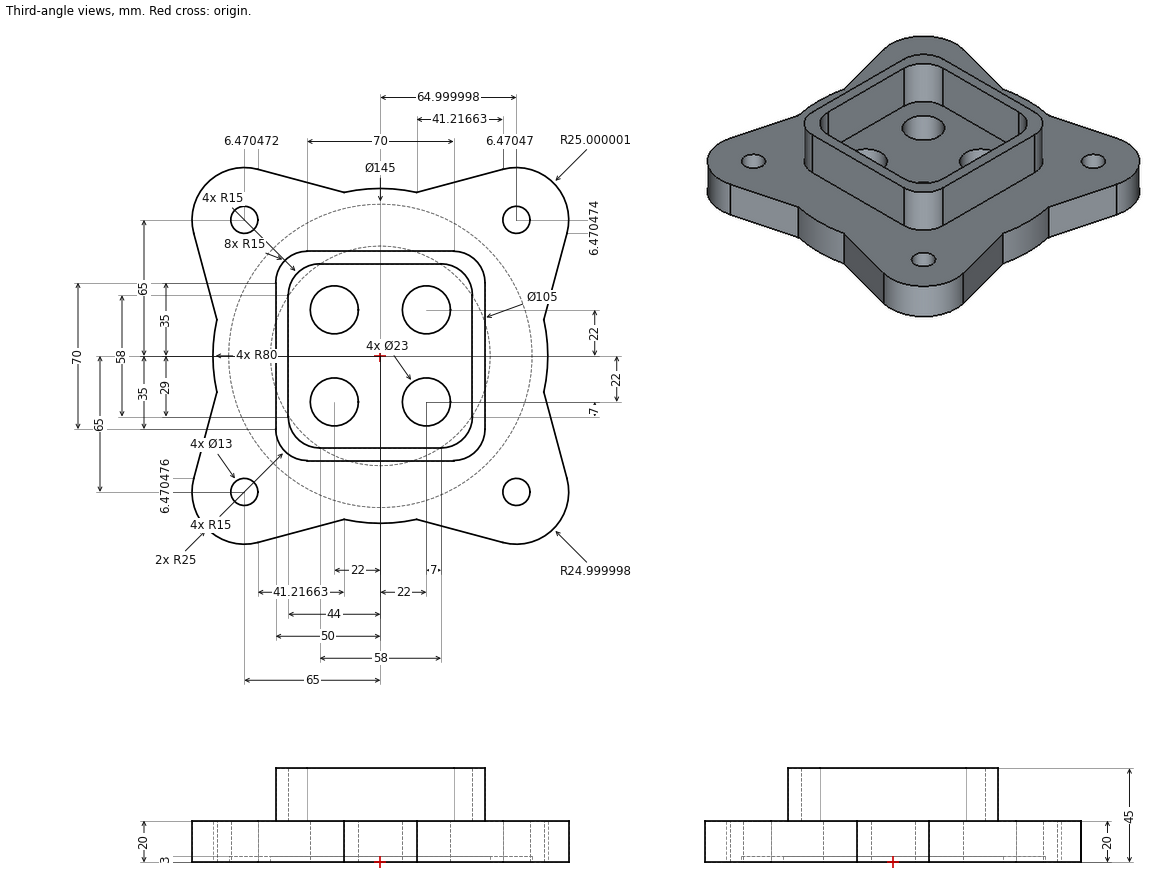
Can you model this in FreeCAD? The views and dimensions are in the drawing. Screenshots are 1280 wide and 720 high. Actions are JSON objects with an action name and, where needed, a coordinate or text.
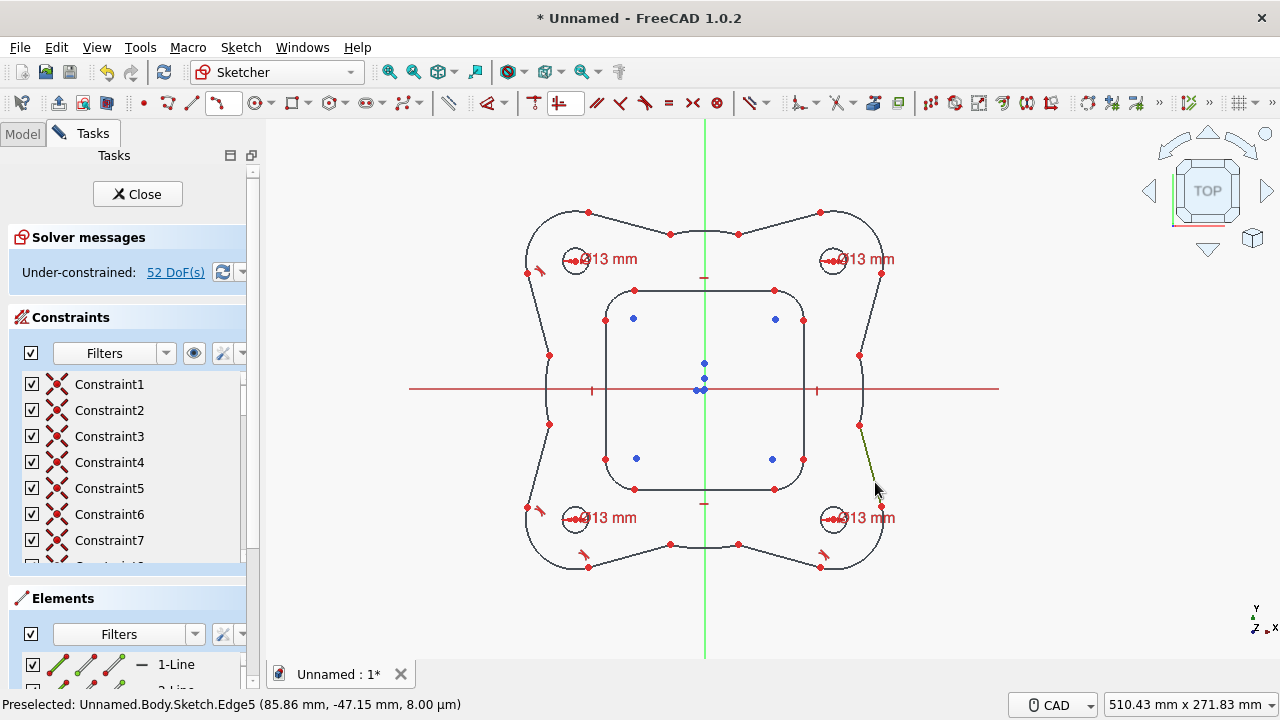
{"action": "left_click", "coordinate": [851, 566]}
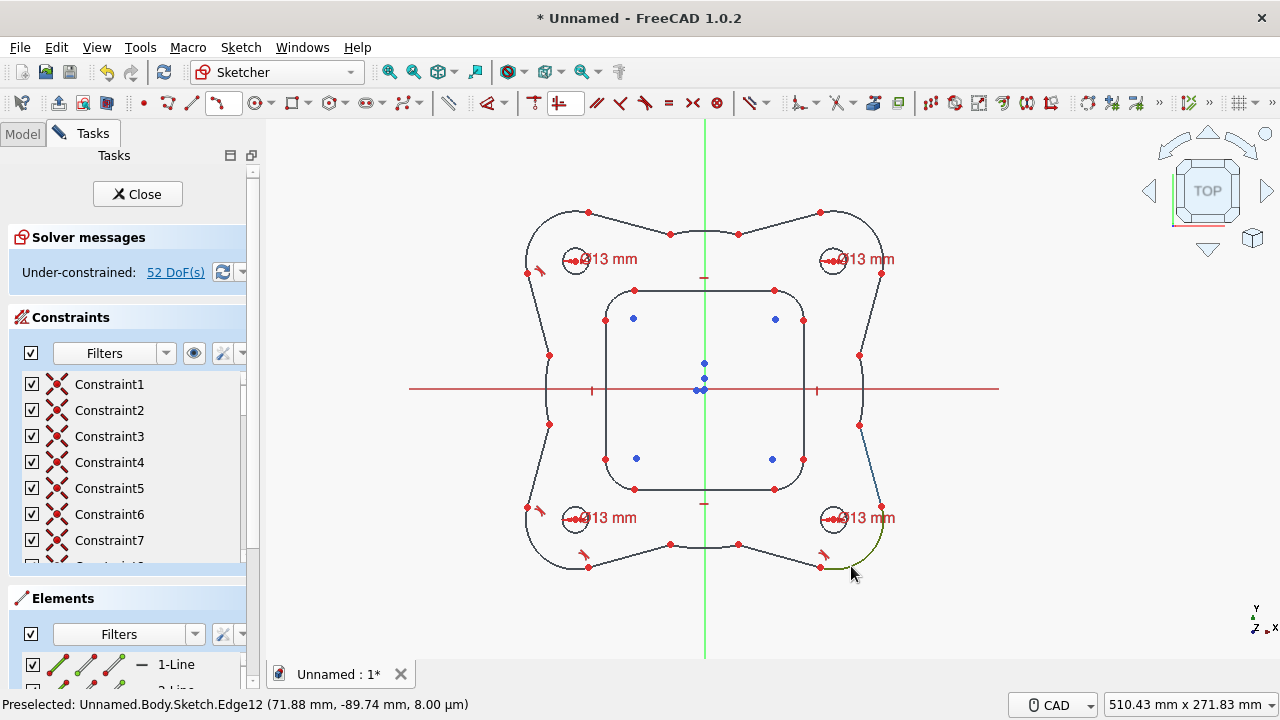
{"action": "left_click", "coordinate": [646, 104]}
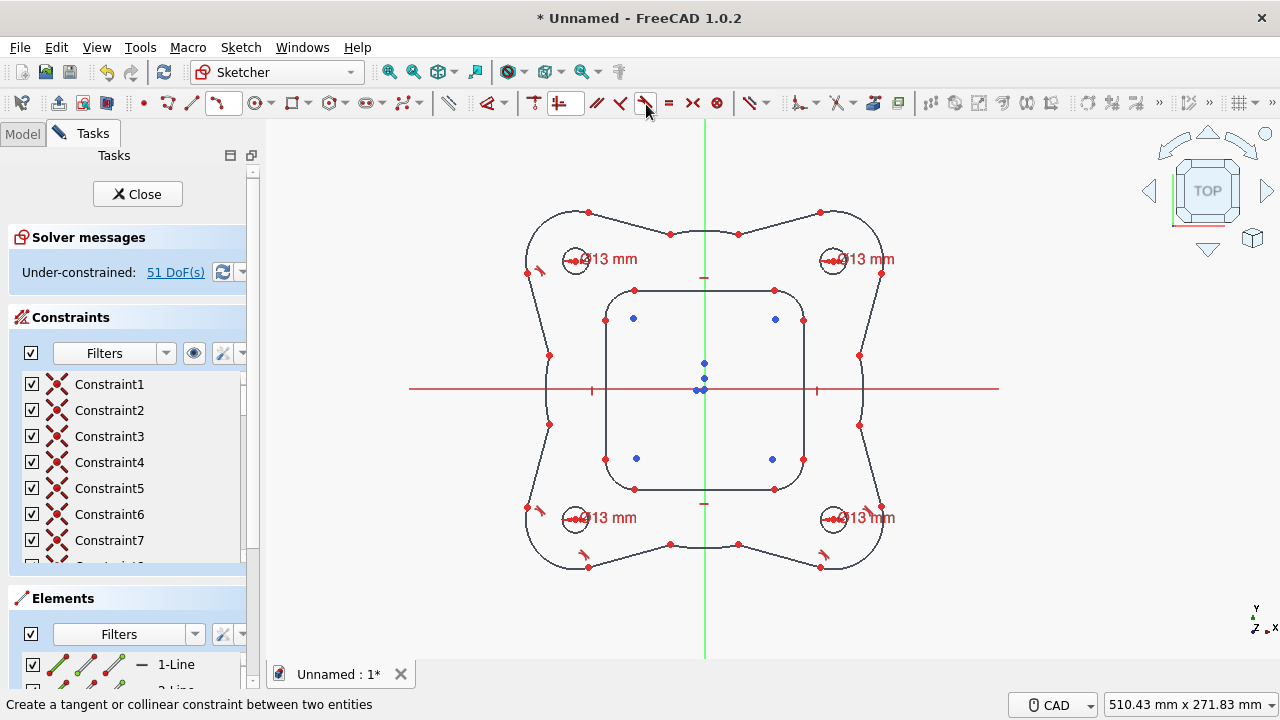
{"action": "left_click", "coordinate": [866, 331]}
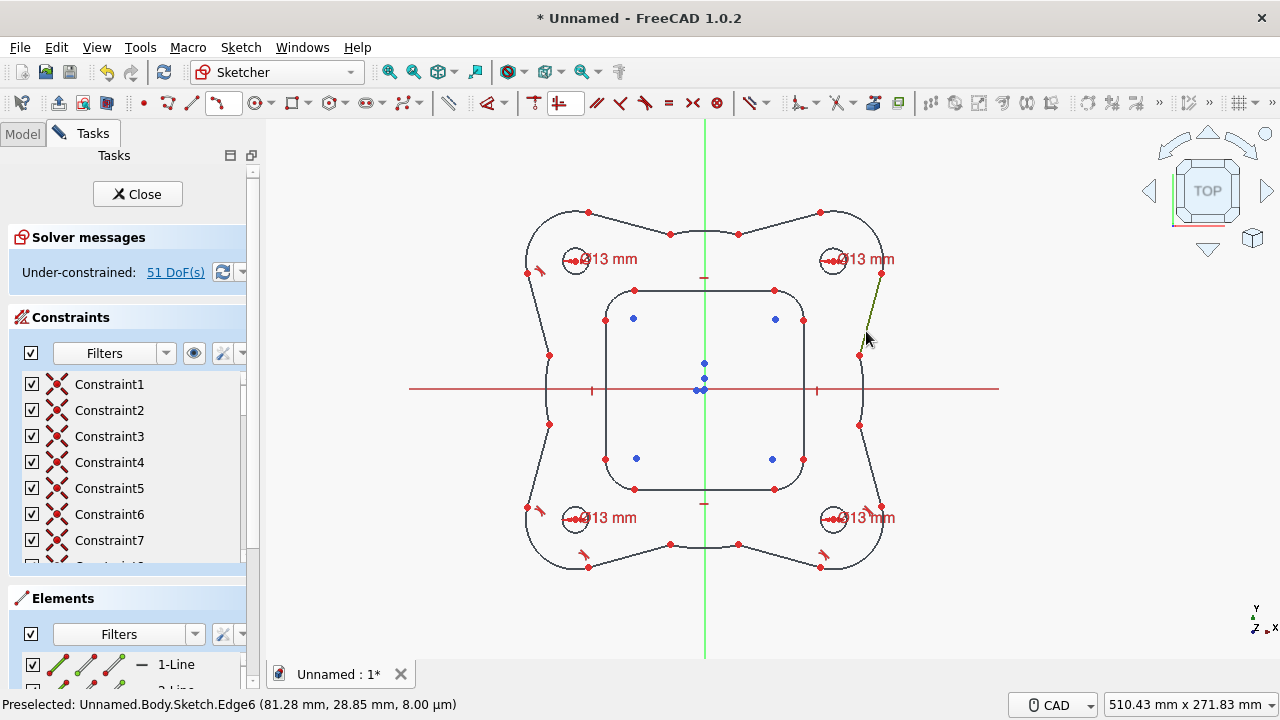
{"action": "left_click", "coordinate": [880, 243]}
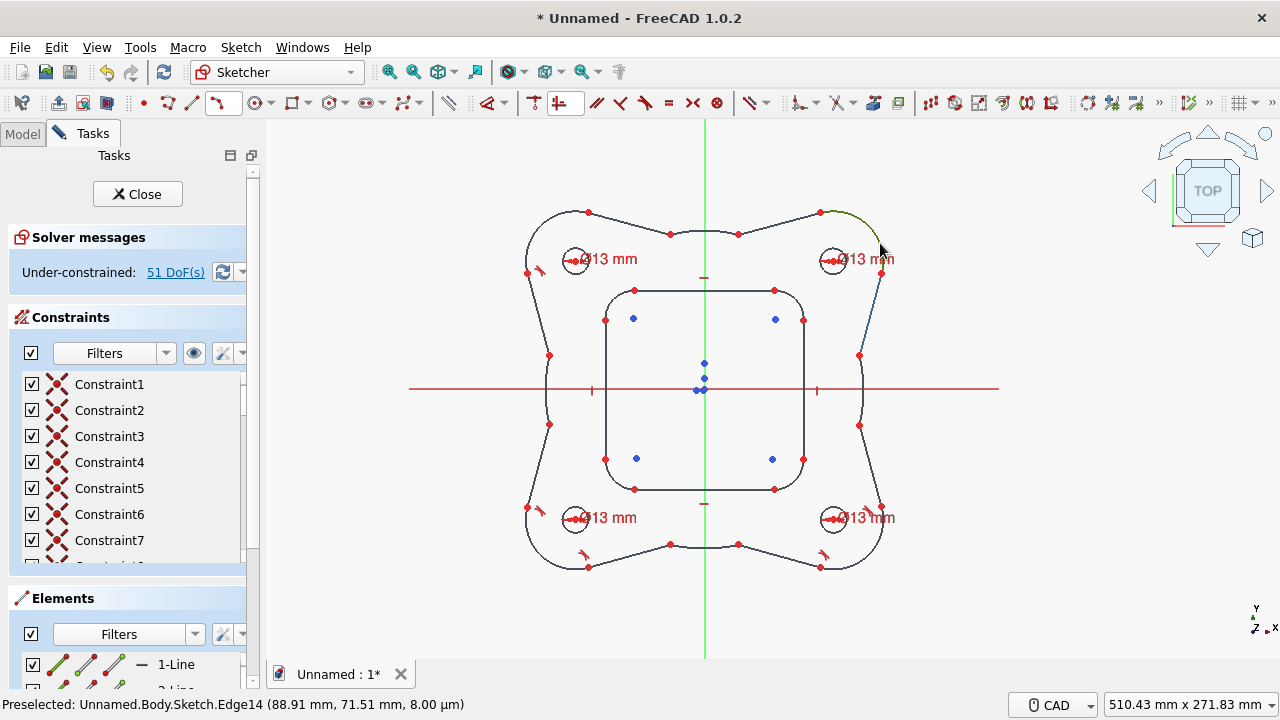
{"action": "left_click", "coordinate": [646, 104]}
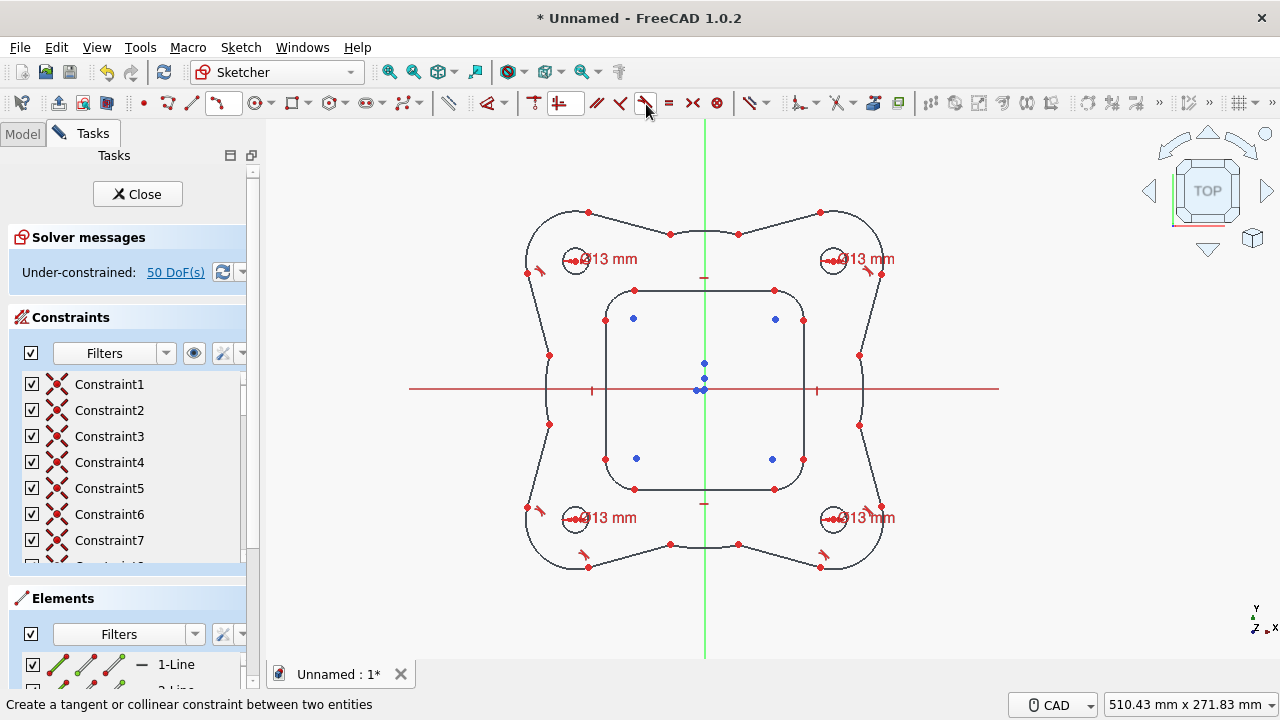
{"action": "left_click", "coordinate": [796, 220]}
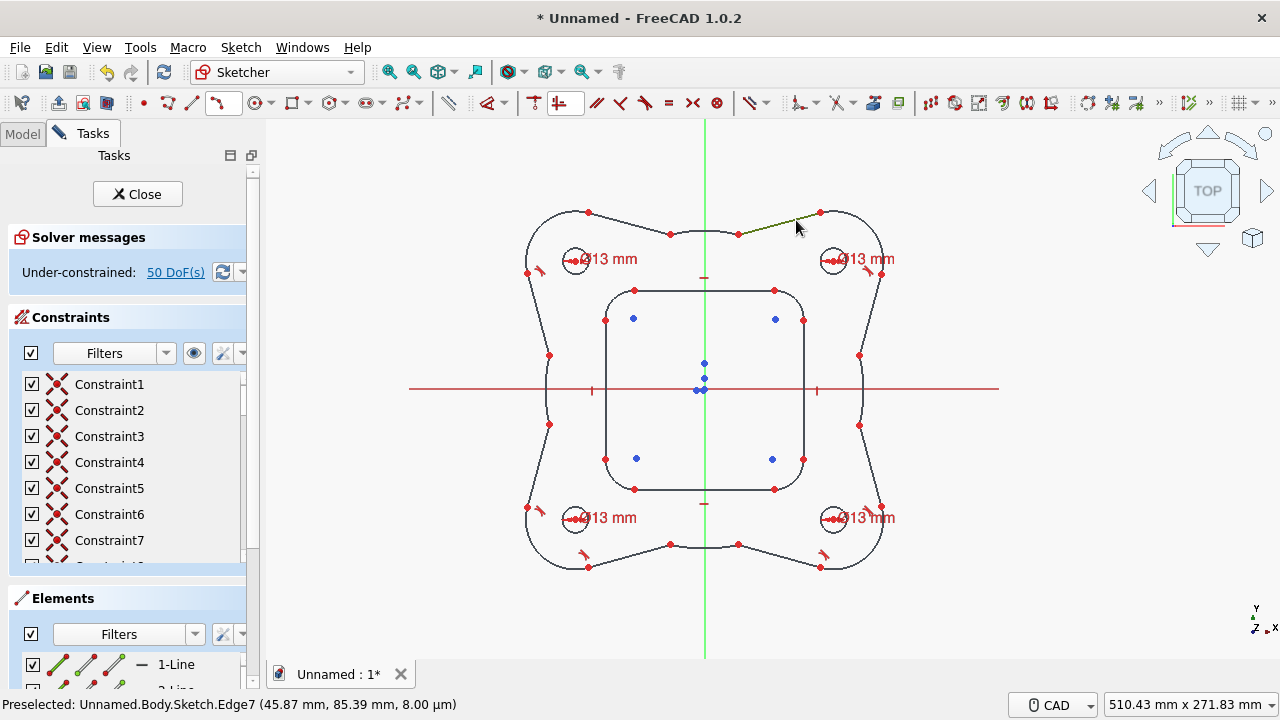
{"action": "left_click", "coordinate": [880, 243]}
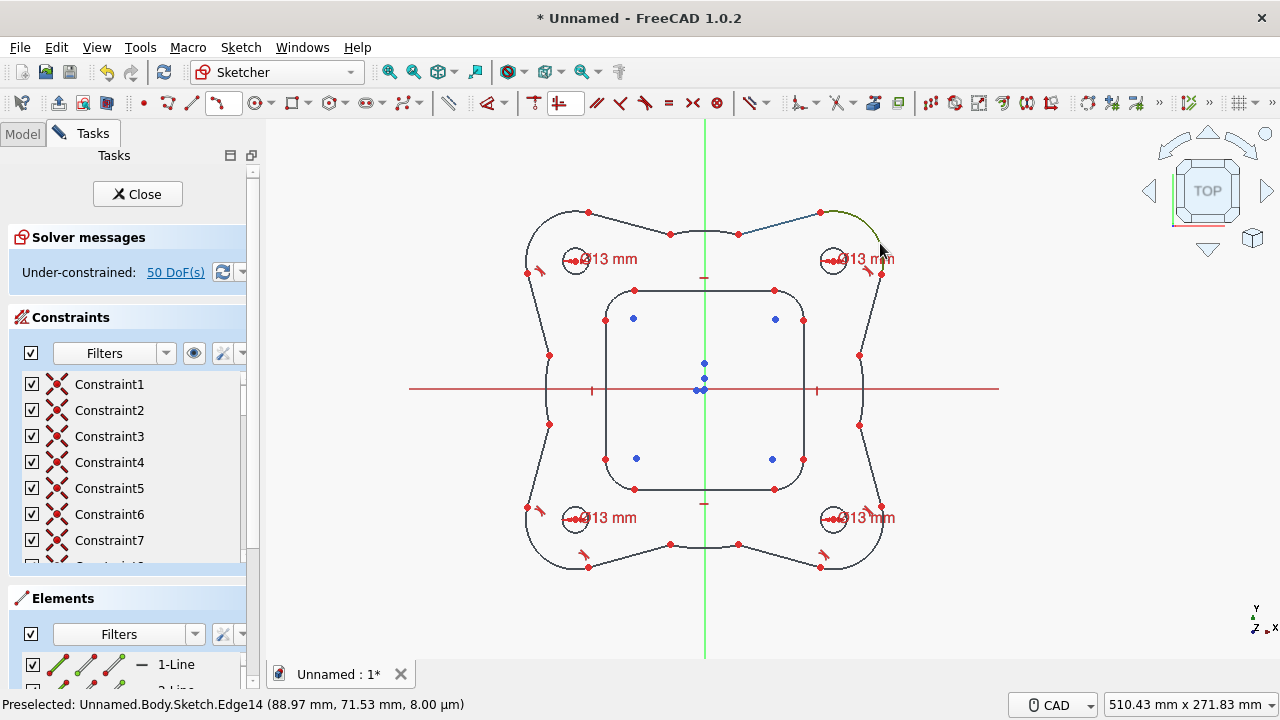
{"action": "left_click", "coordinate": [646, 104]}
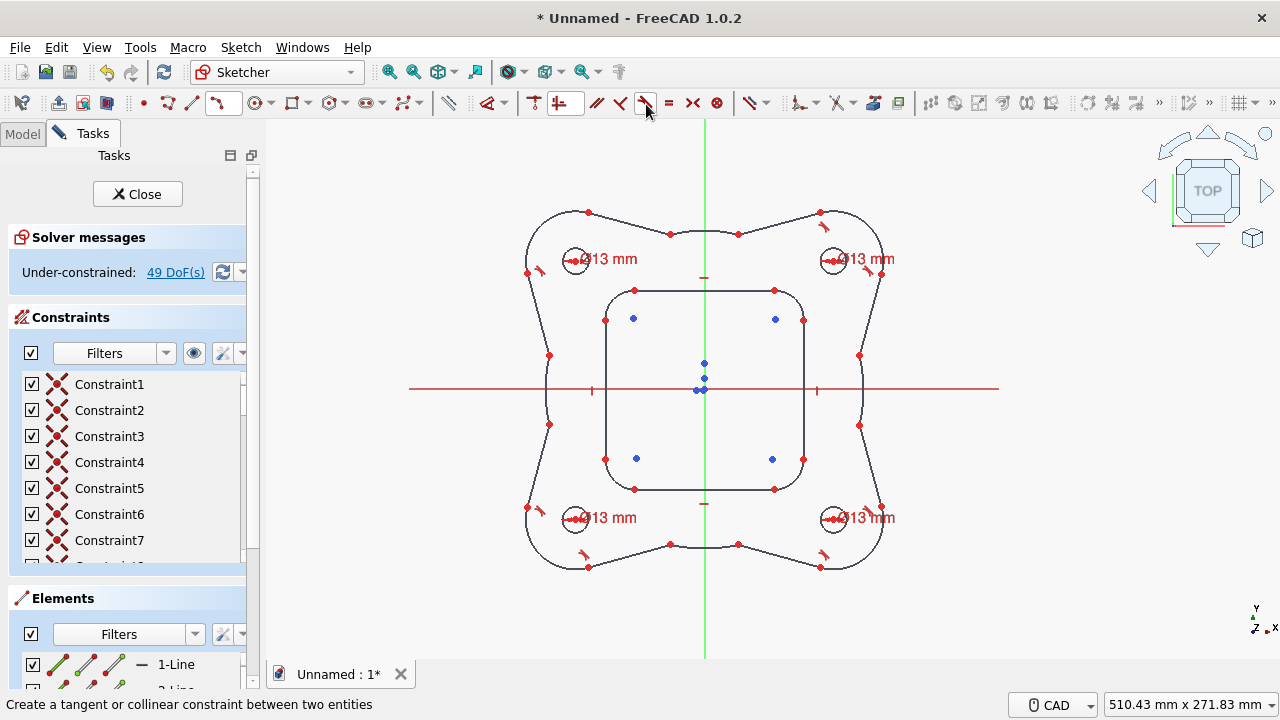
{"action": "left_click", "coordinate": [646, 228]}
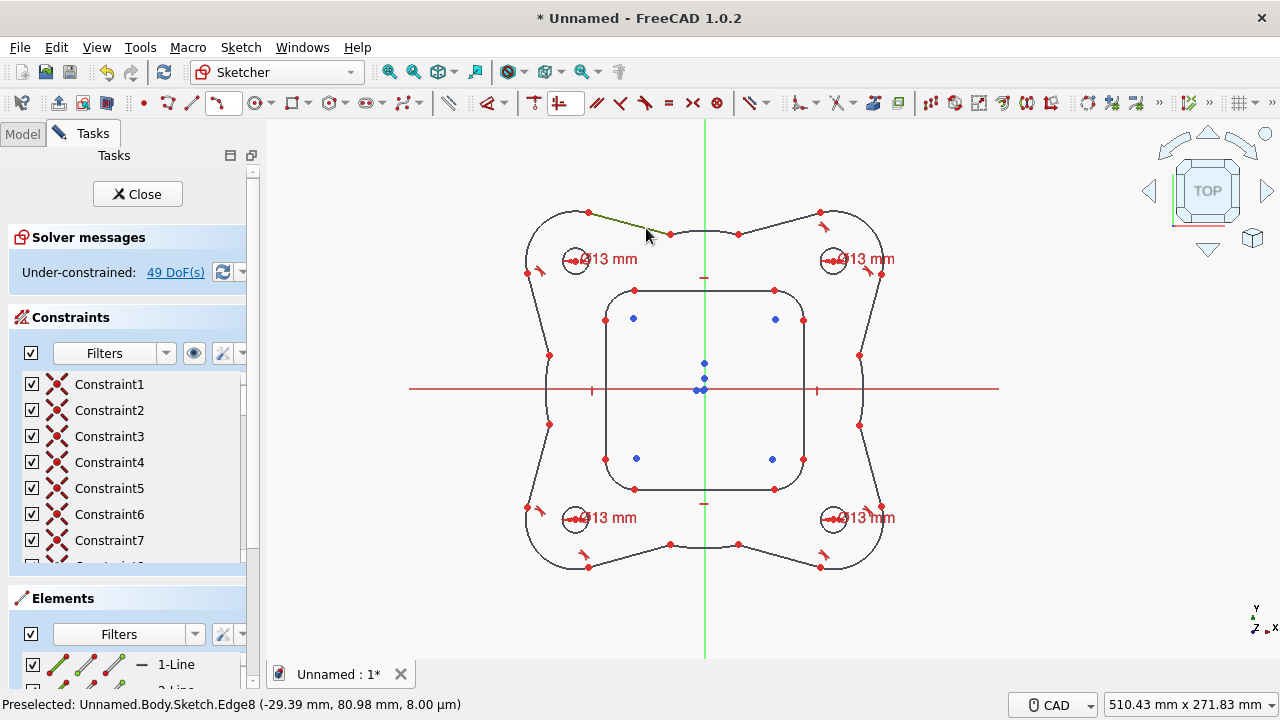
{"action": "left_click", "coordinate": [558, 215]}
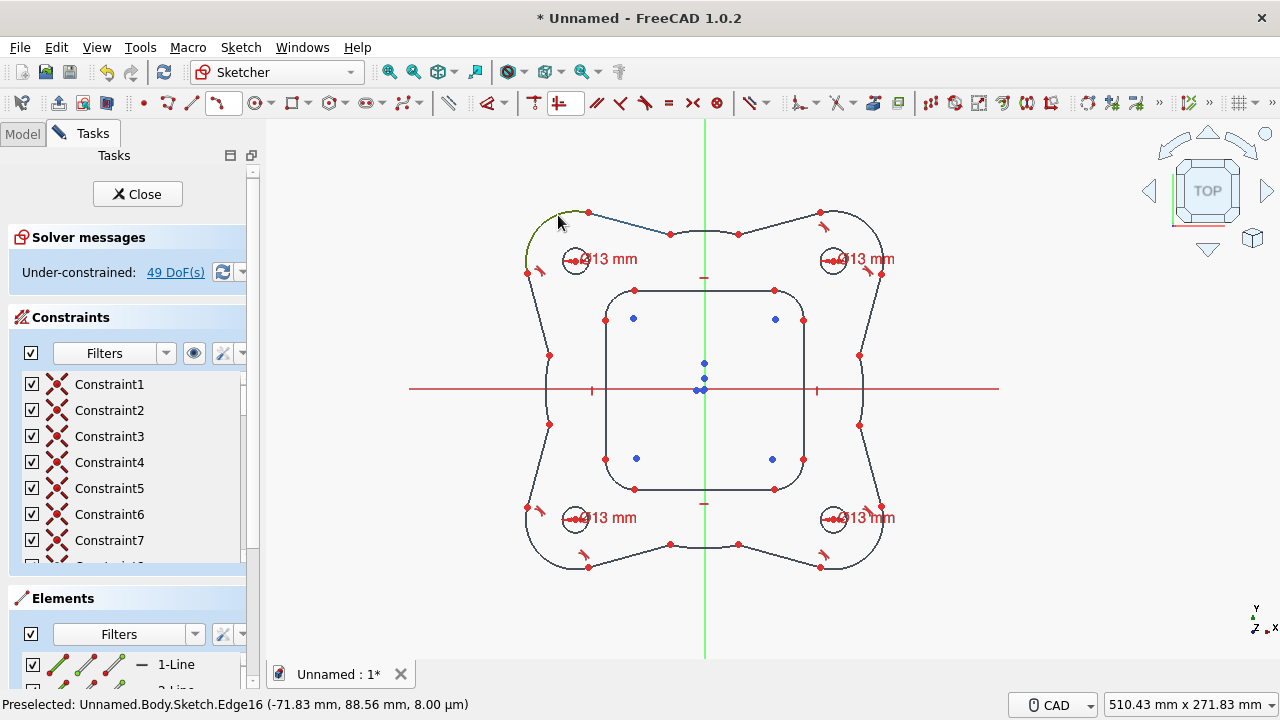
{"action": "left_click", "coordinate": [646, 104]}